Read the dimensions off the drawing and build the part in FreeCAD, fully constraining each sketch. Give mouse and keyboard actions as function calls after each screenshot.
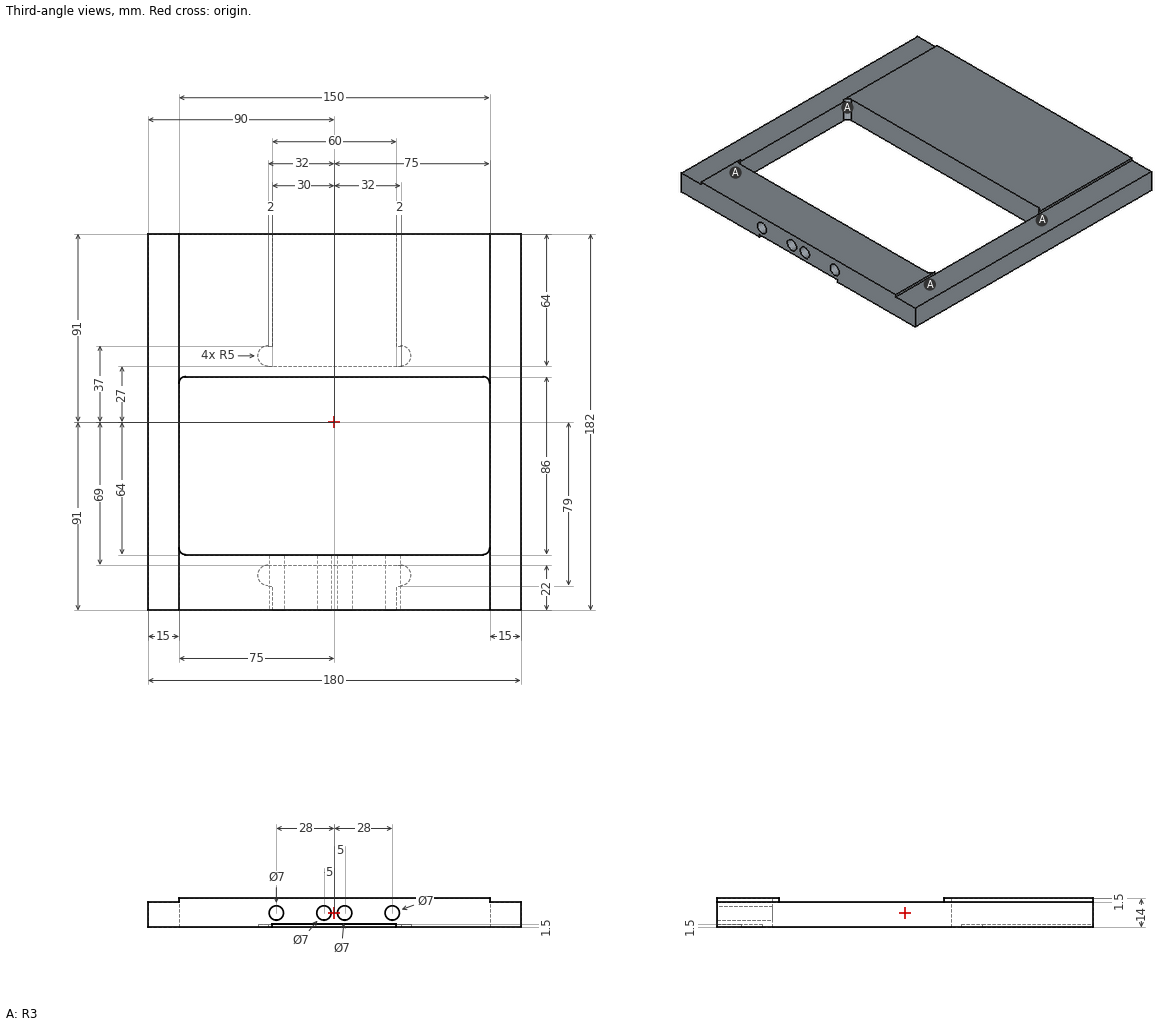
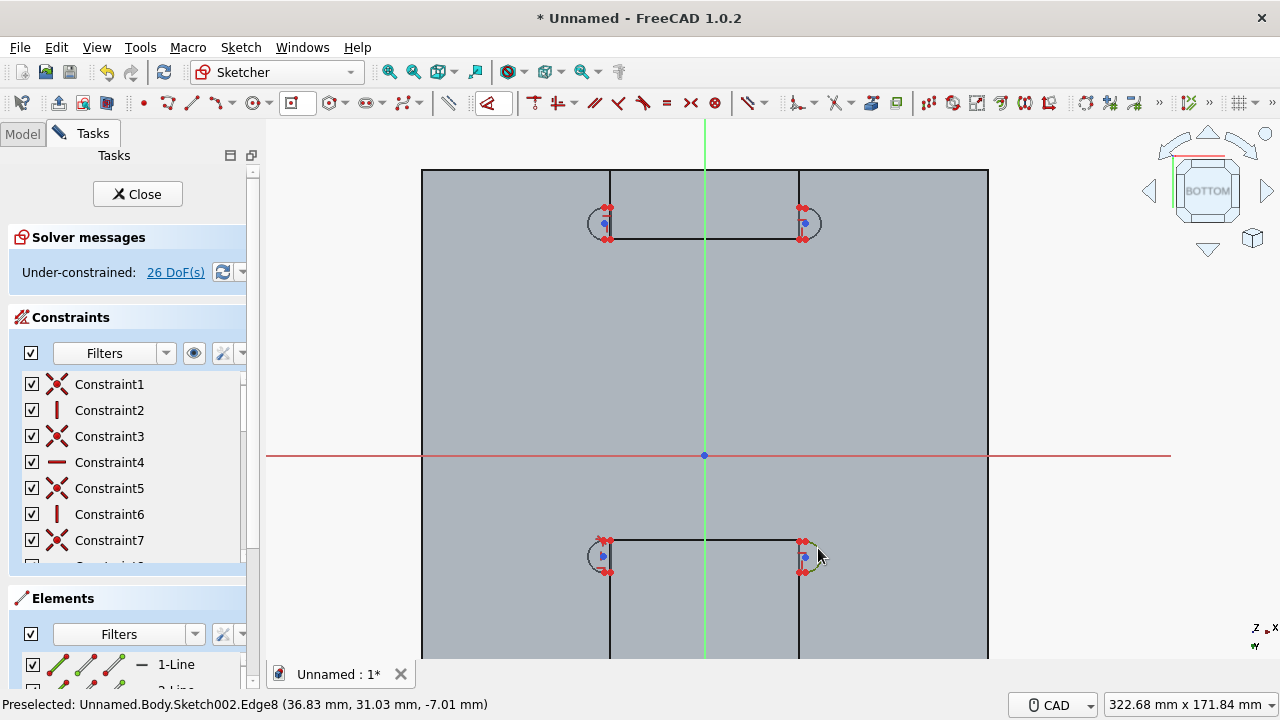
click(644, 104)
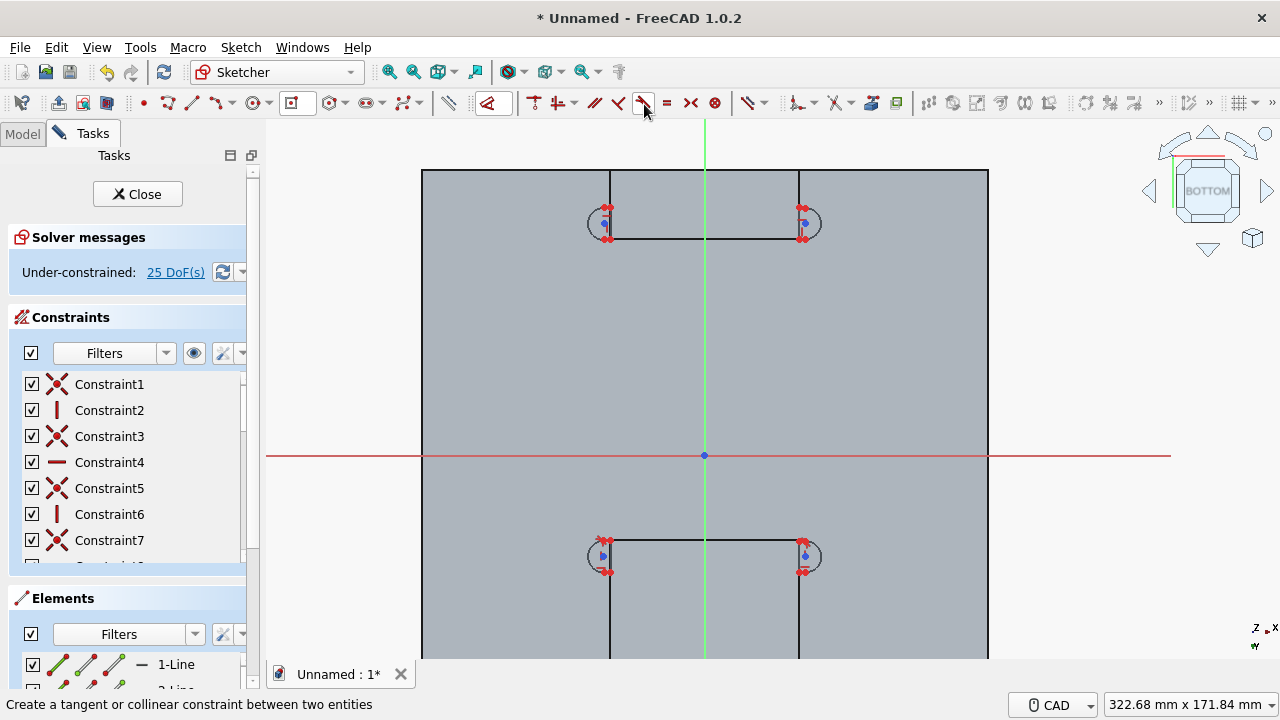
scroll(802, 572, up, 8)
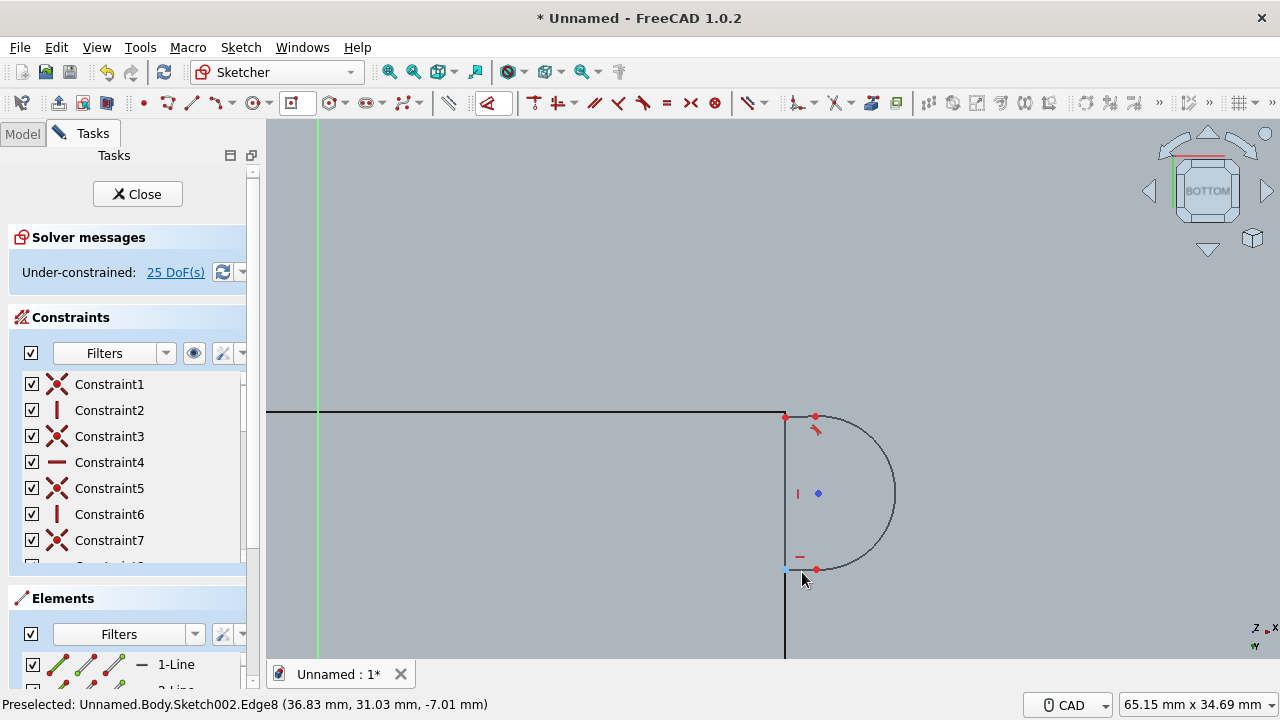
click(801, 570)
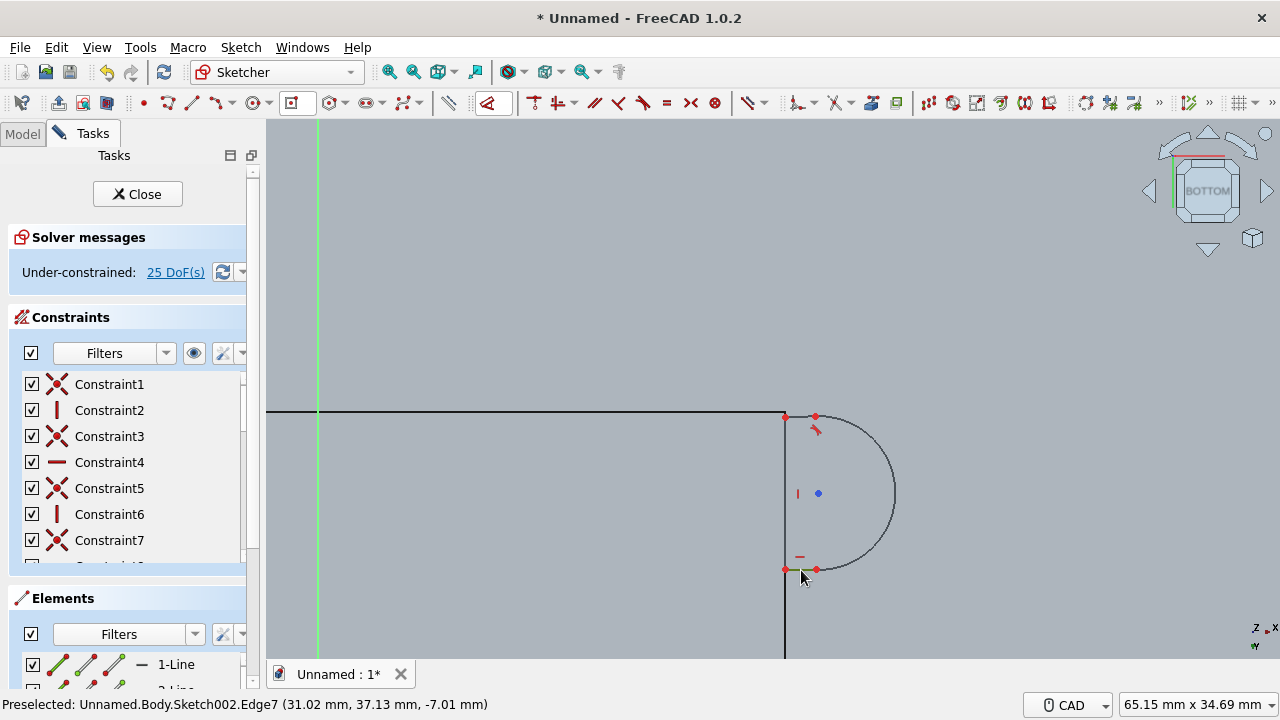
scroll(802, 572, down, 8)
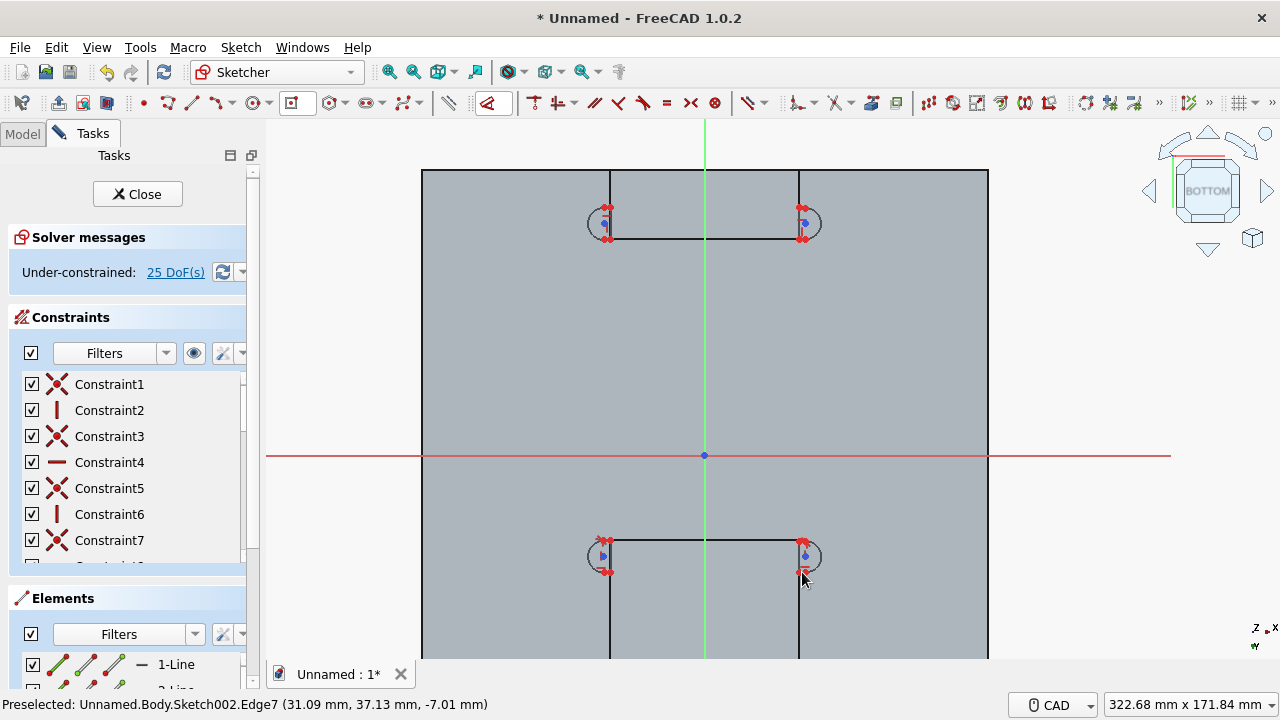
click(818, 566)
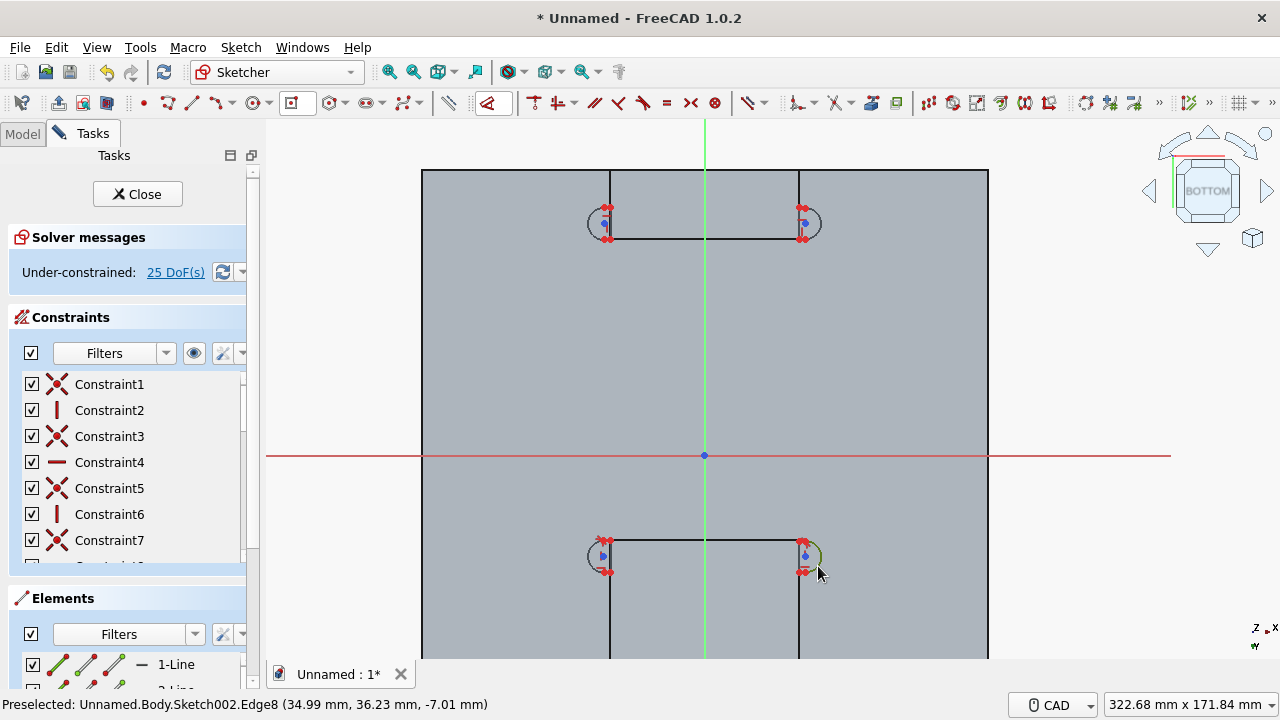
key(t)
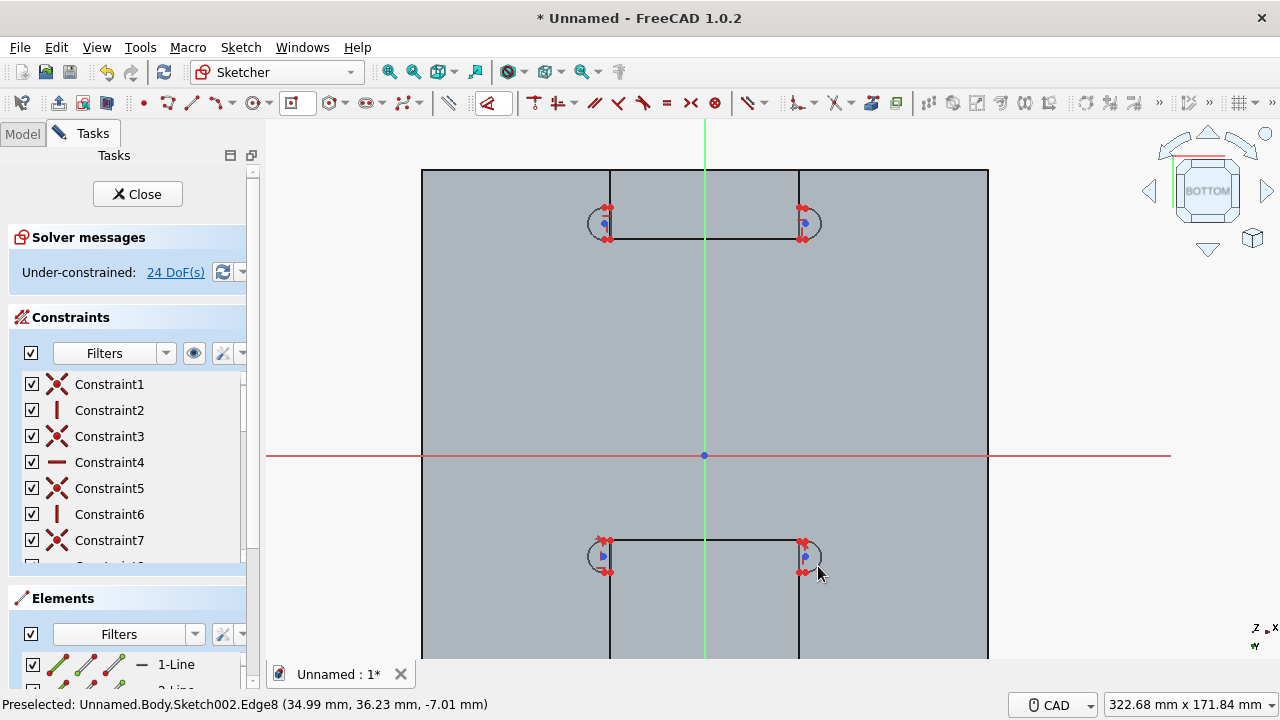
scroll(607, 240, up, 8)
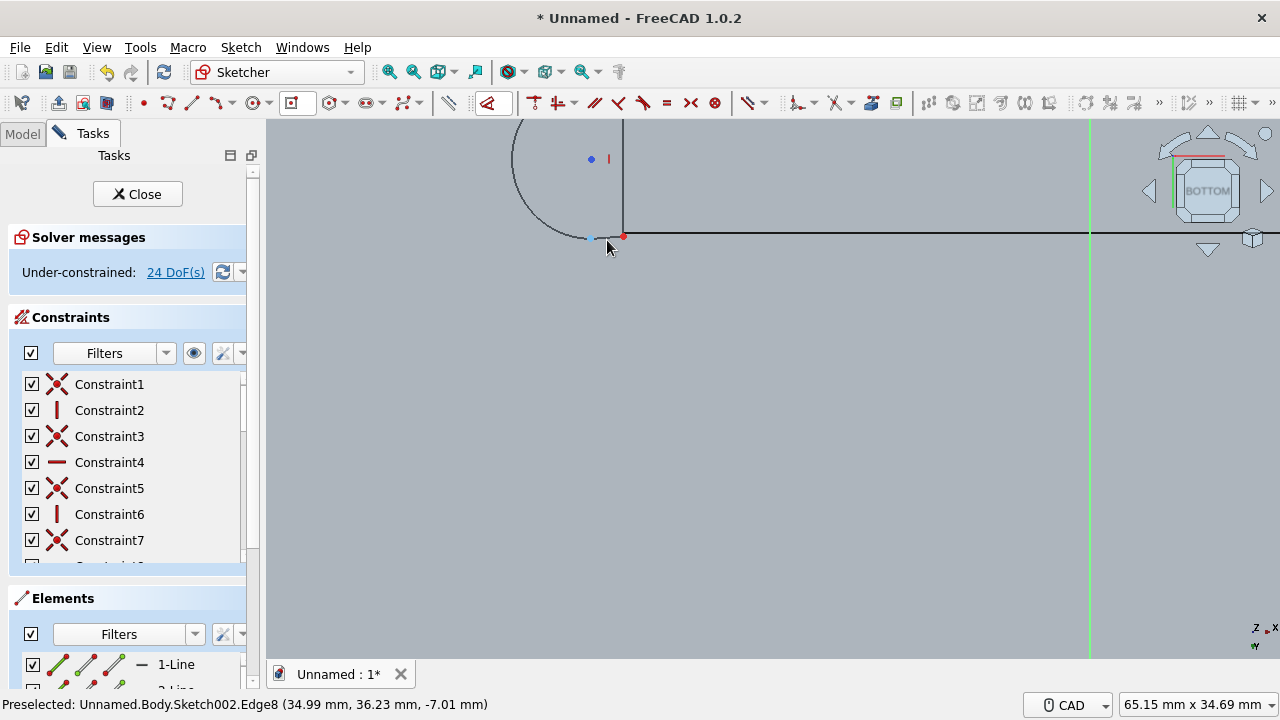
click(607, 238)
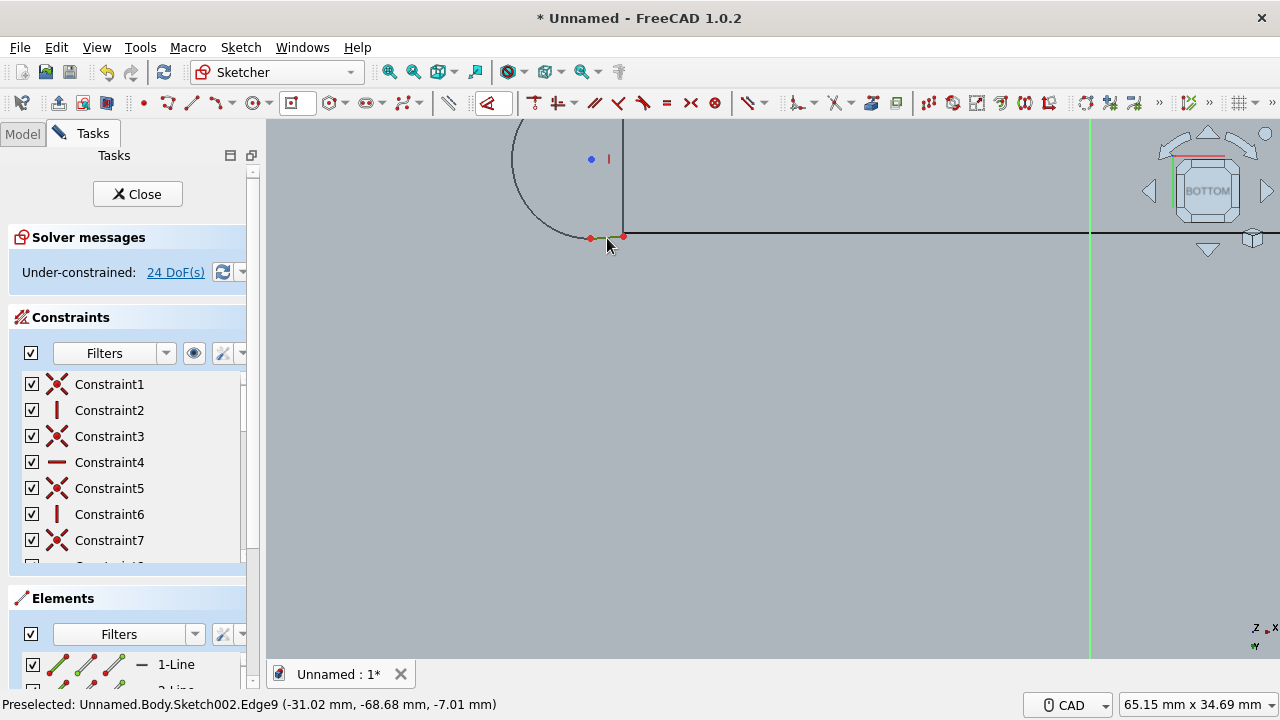
scroll(607, 240, down, 8)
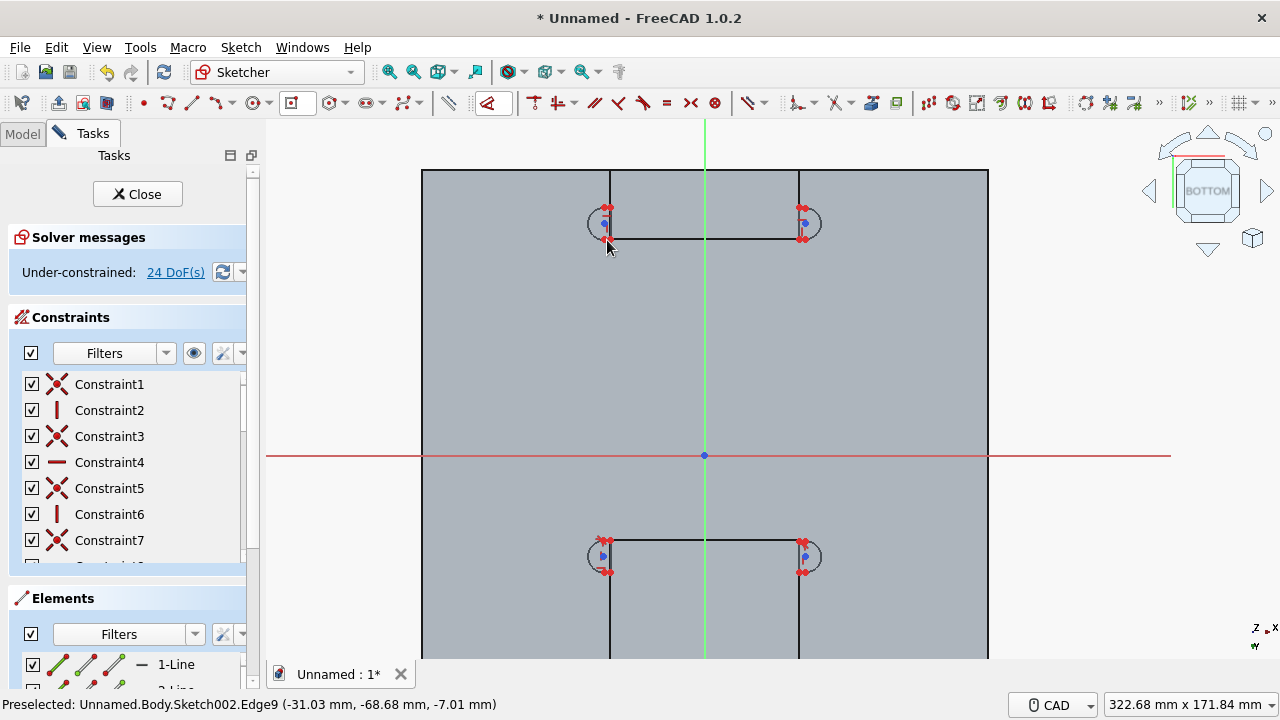
click(591, 233)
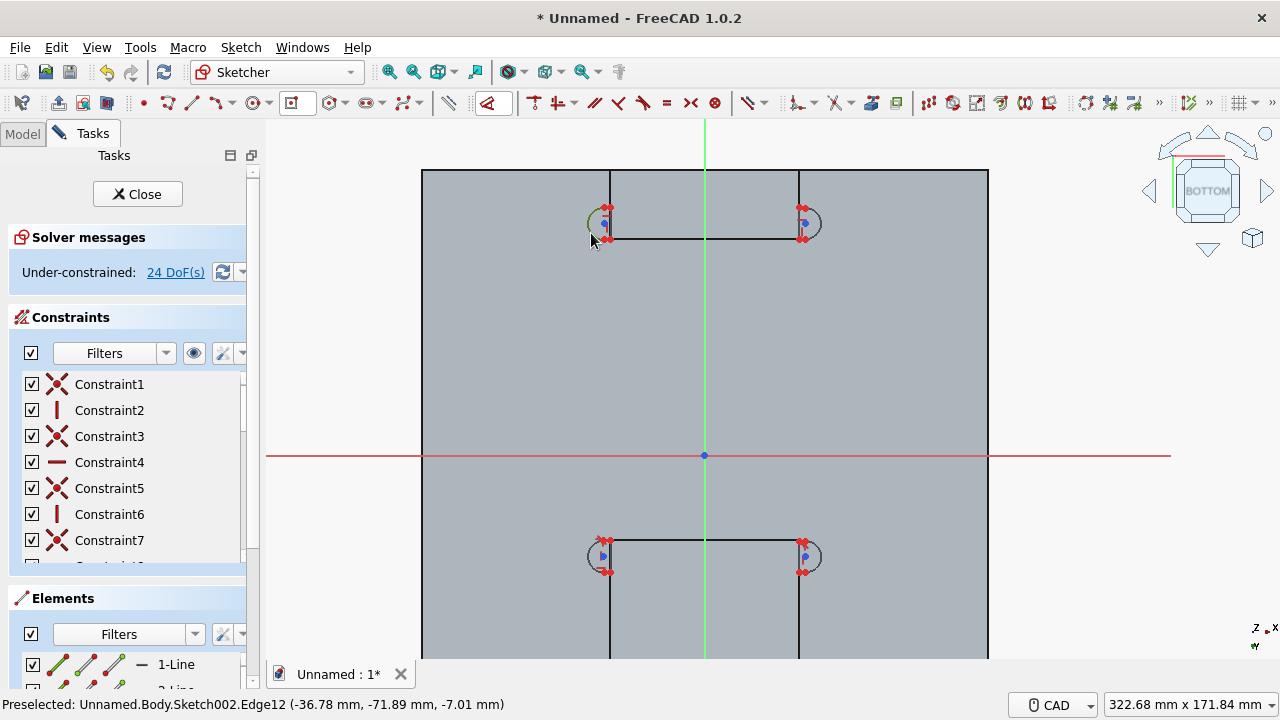
key(t)